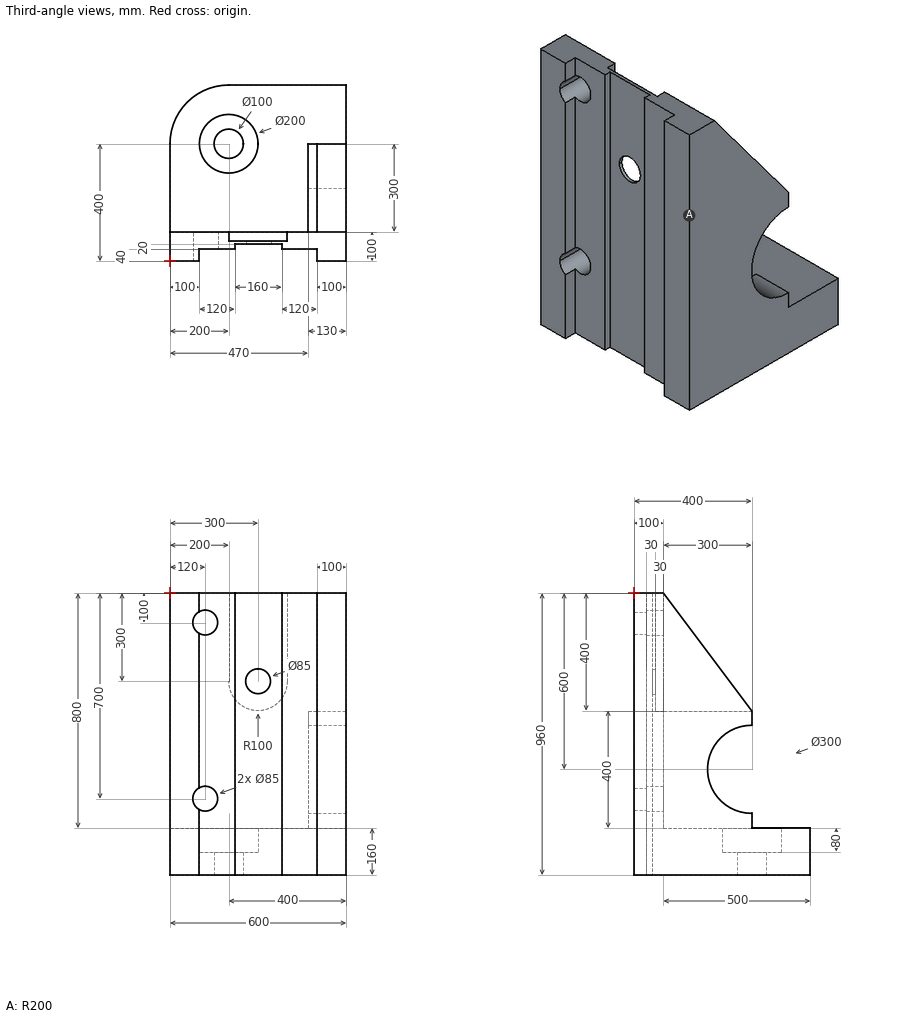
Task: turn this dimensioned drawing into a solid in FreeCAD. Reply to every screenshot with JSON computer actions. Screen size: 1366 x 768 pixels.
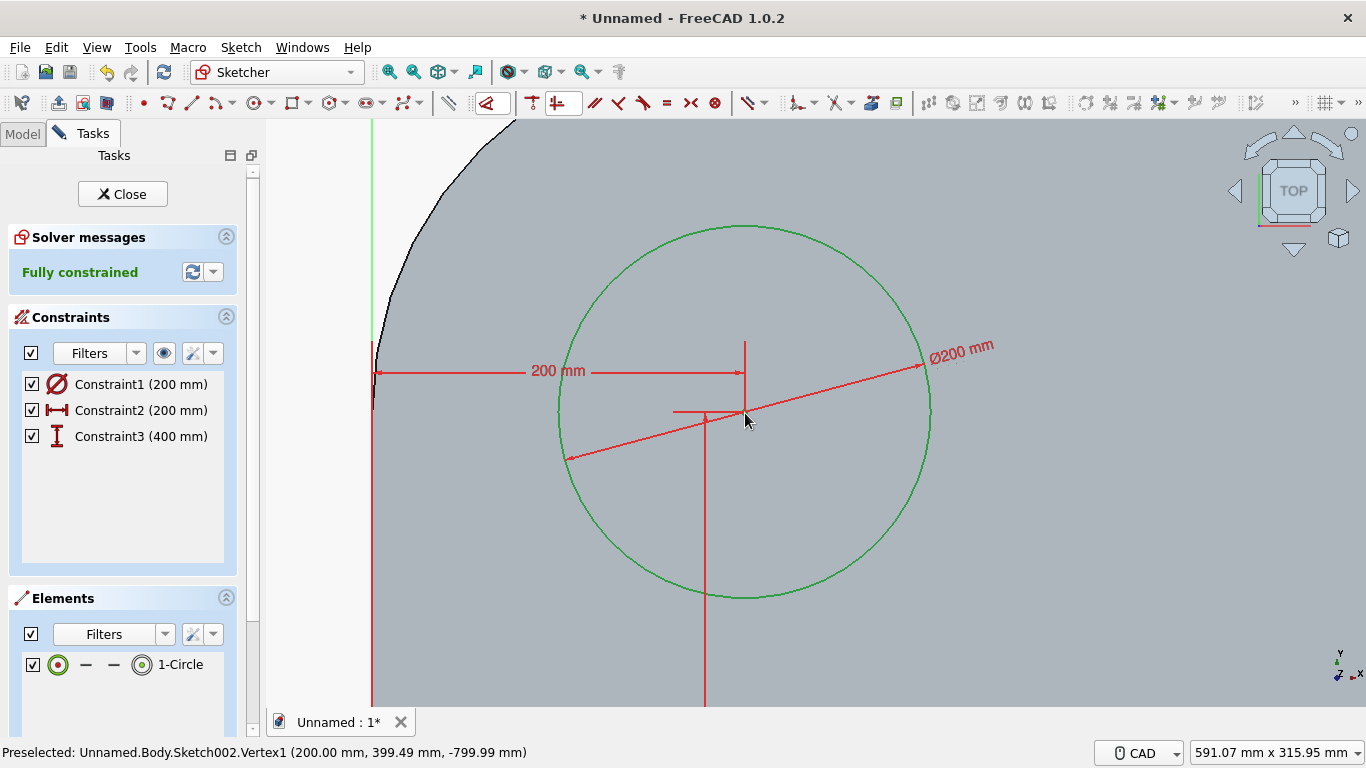
{"action": "left_click", "coordinate": [123, 194]}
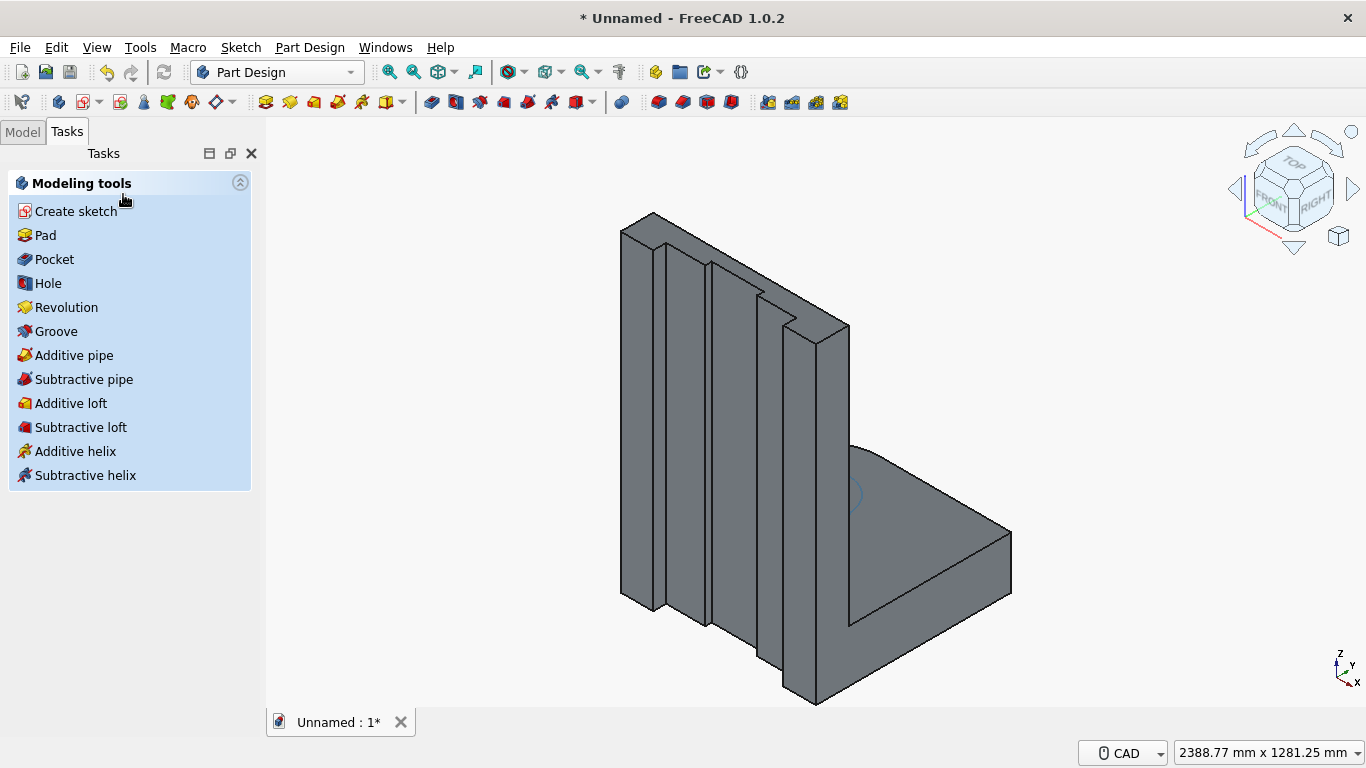
{"action": "left_click", "coordinate": [432, 102]}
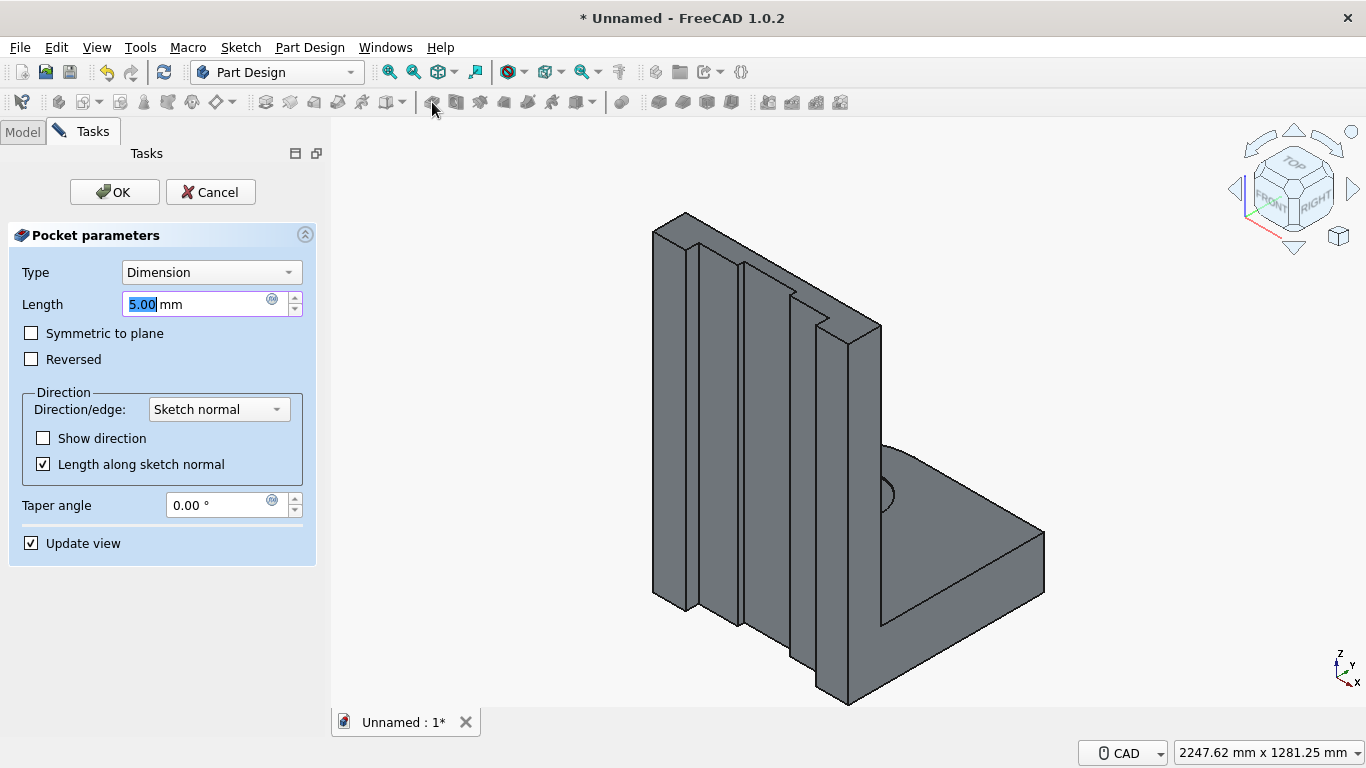
{"action": "type", "text": "80"}
{"action": "key", "text": "Tab"}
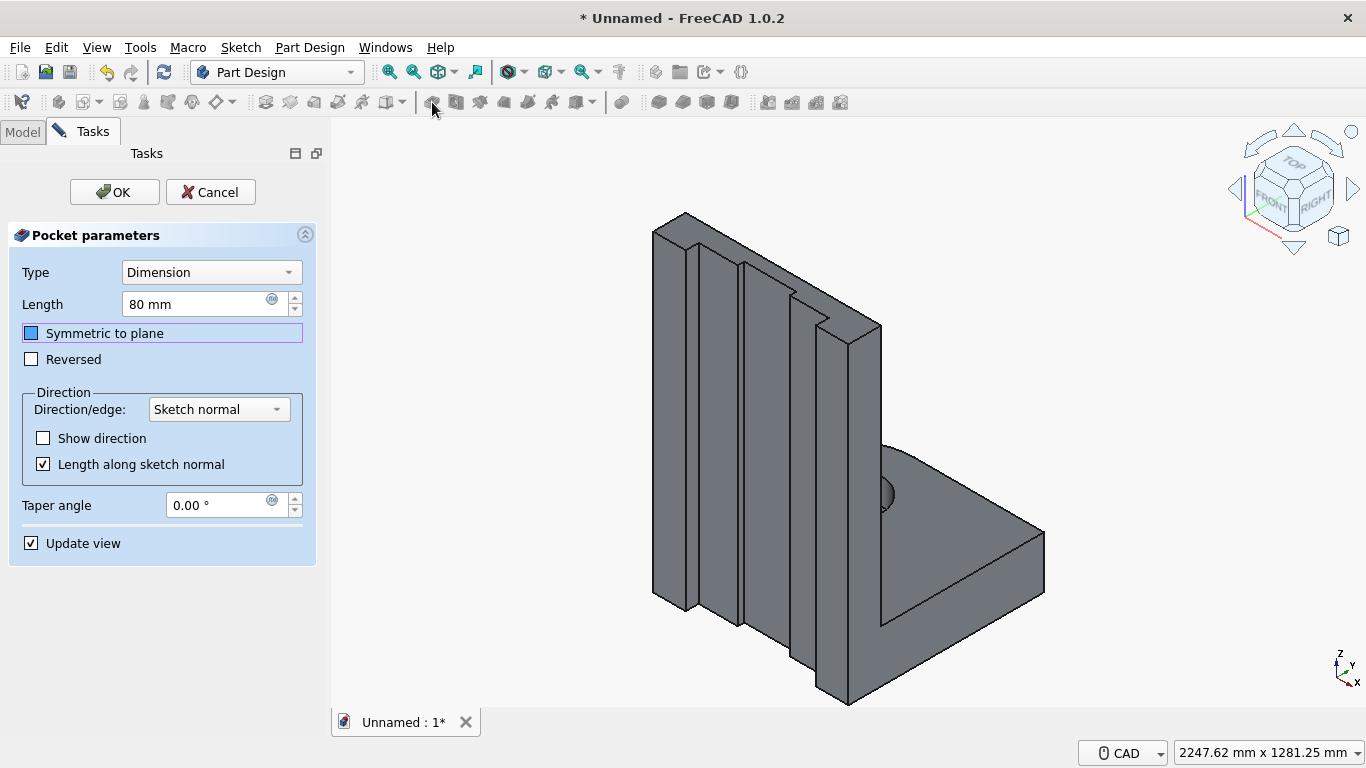
{"action": "left_click", "coordinate": [115, 192]}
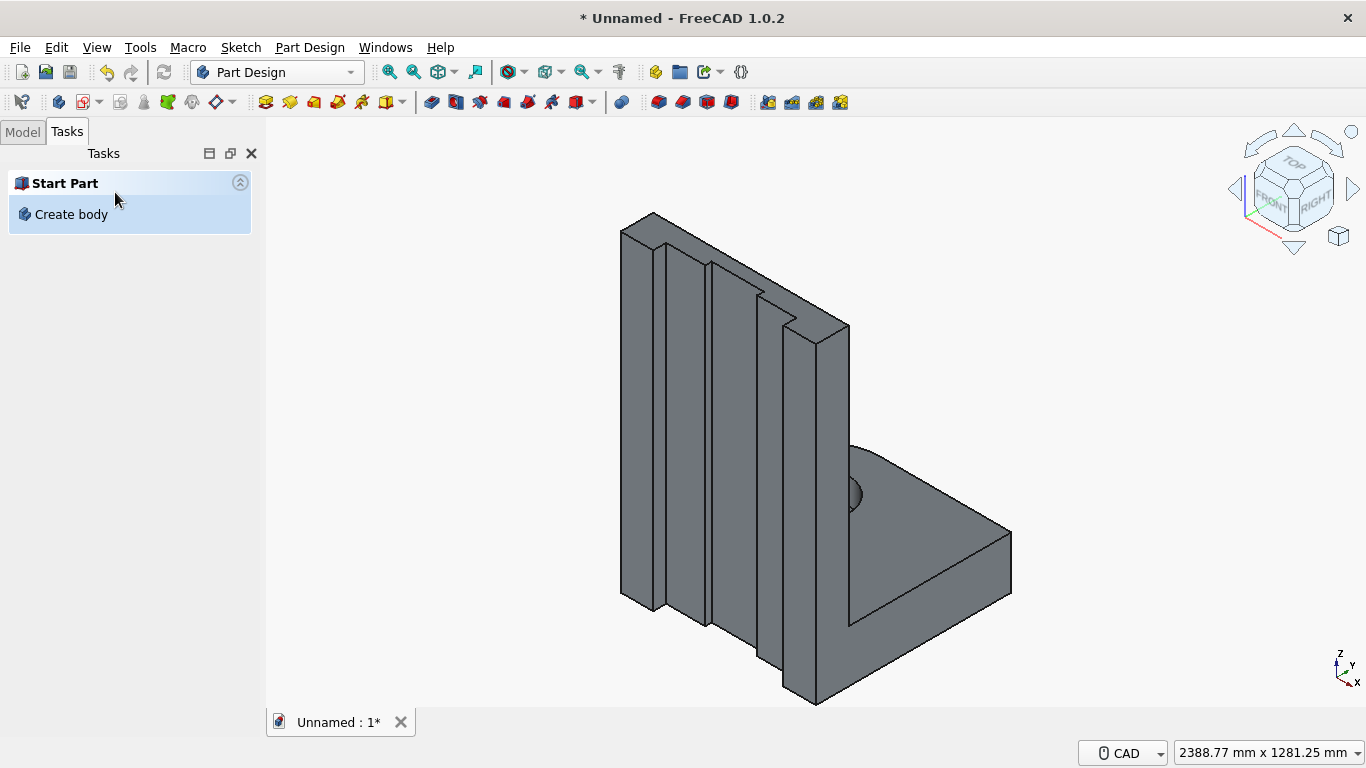
{"action": "key", "text": "2"}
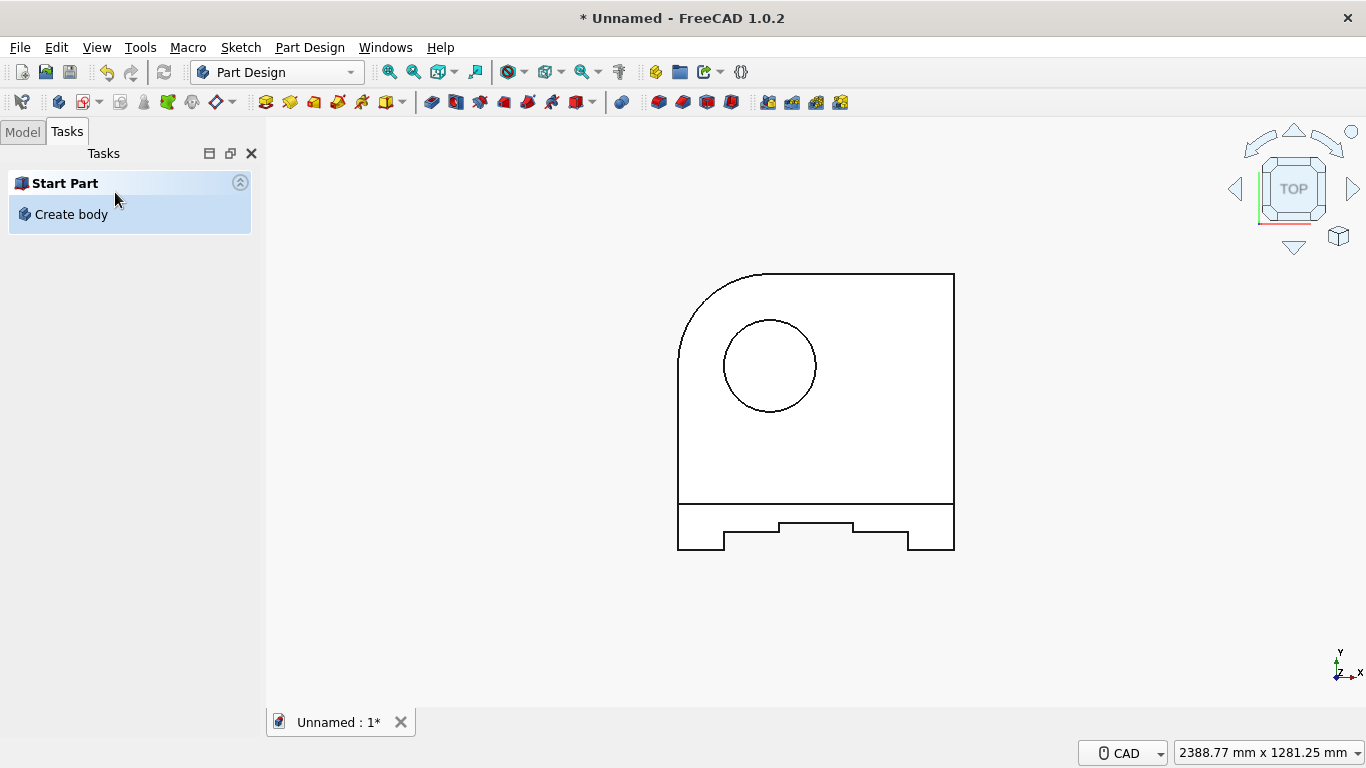
{"action": "left_click", "coordinate": [770, 365]}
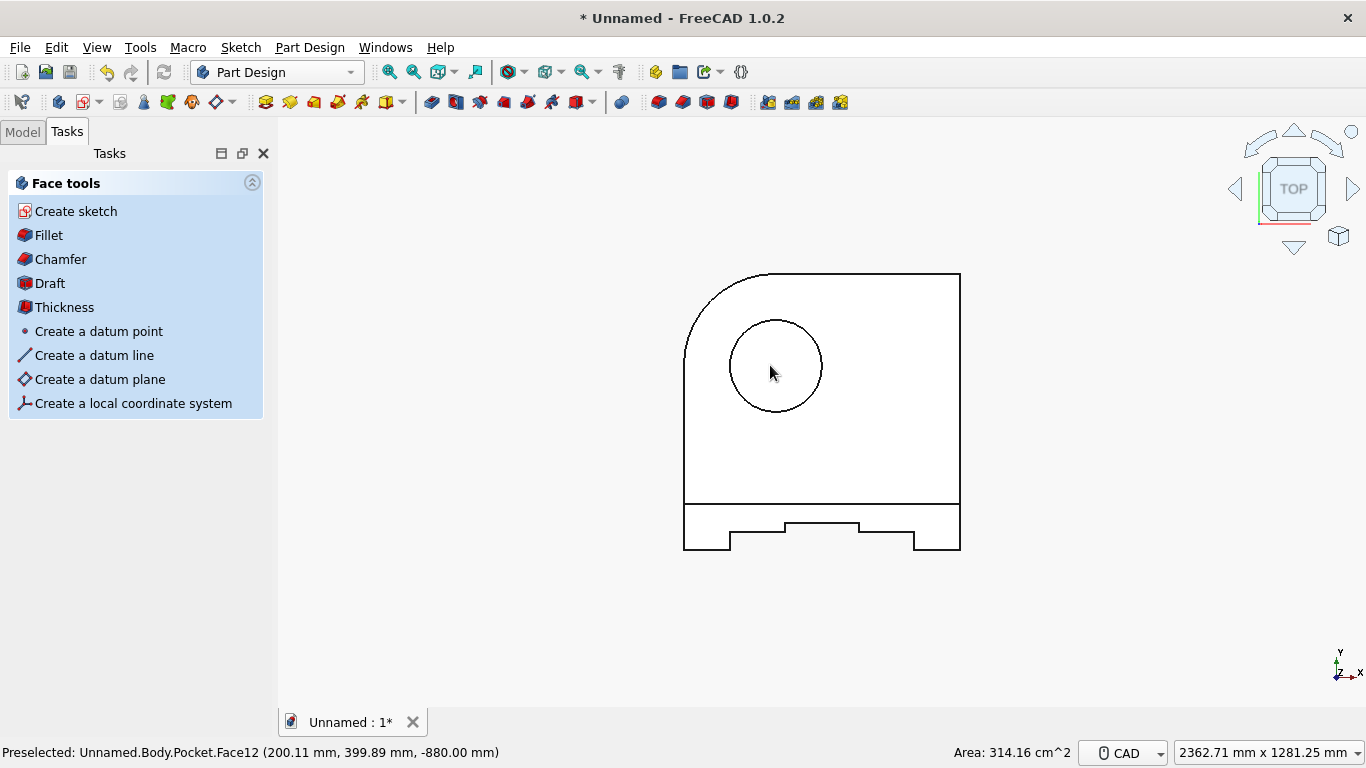
{"action": "left_click", "coordinate": [84, 102]}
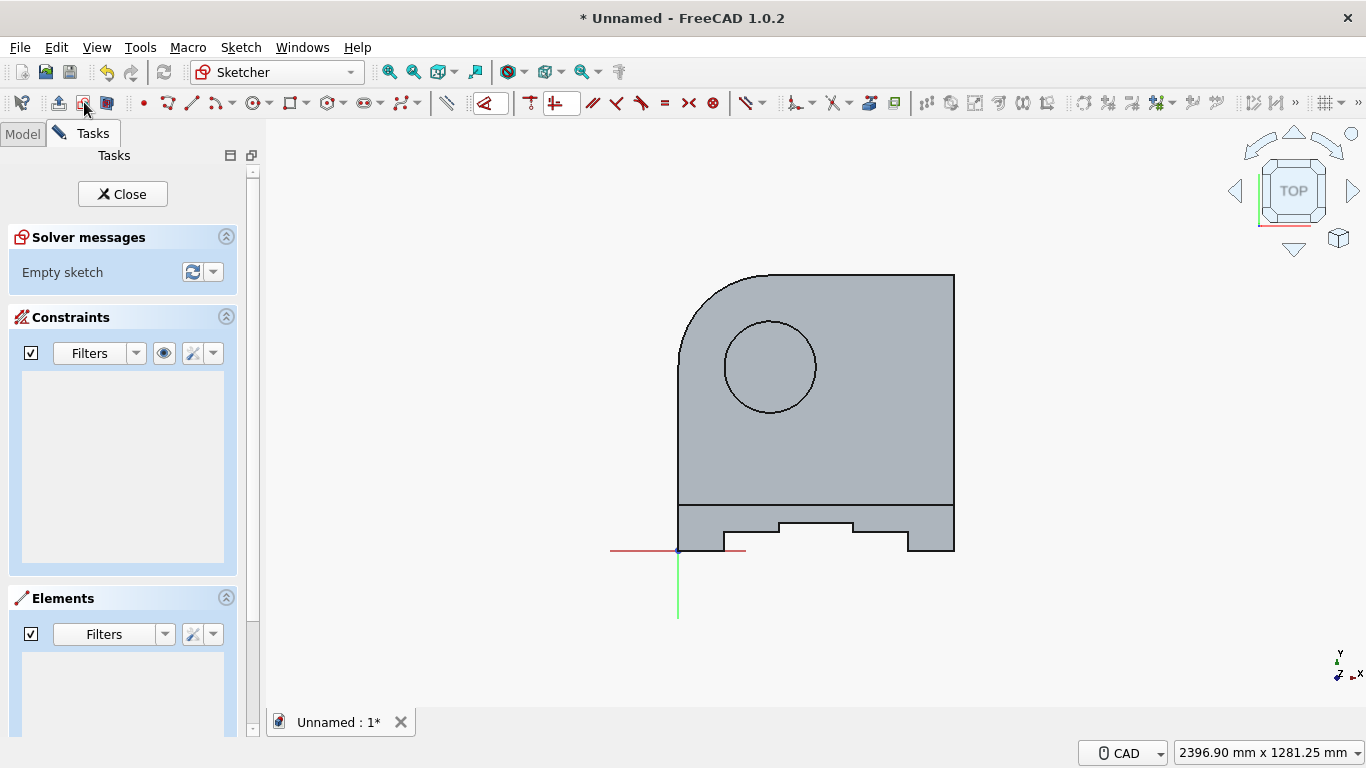
{"action": "left_click", "coordinate": [108, 104]}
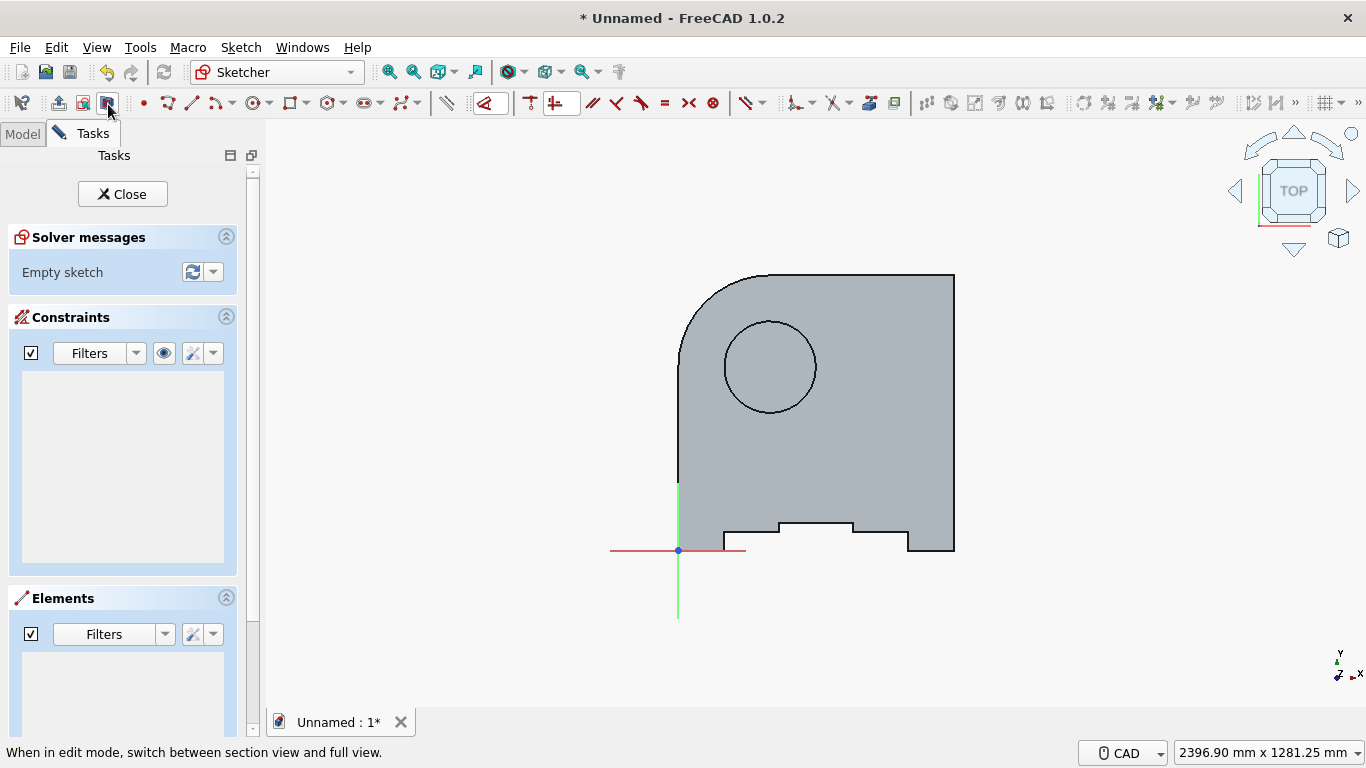
{"action": "scroll", "coordinate": [773, 361], "scroll_direction": "up", "scroll_amount": 11}